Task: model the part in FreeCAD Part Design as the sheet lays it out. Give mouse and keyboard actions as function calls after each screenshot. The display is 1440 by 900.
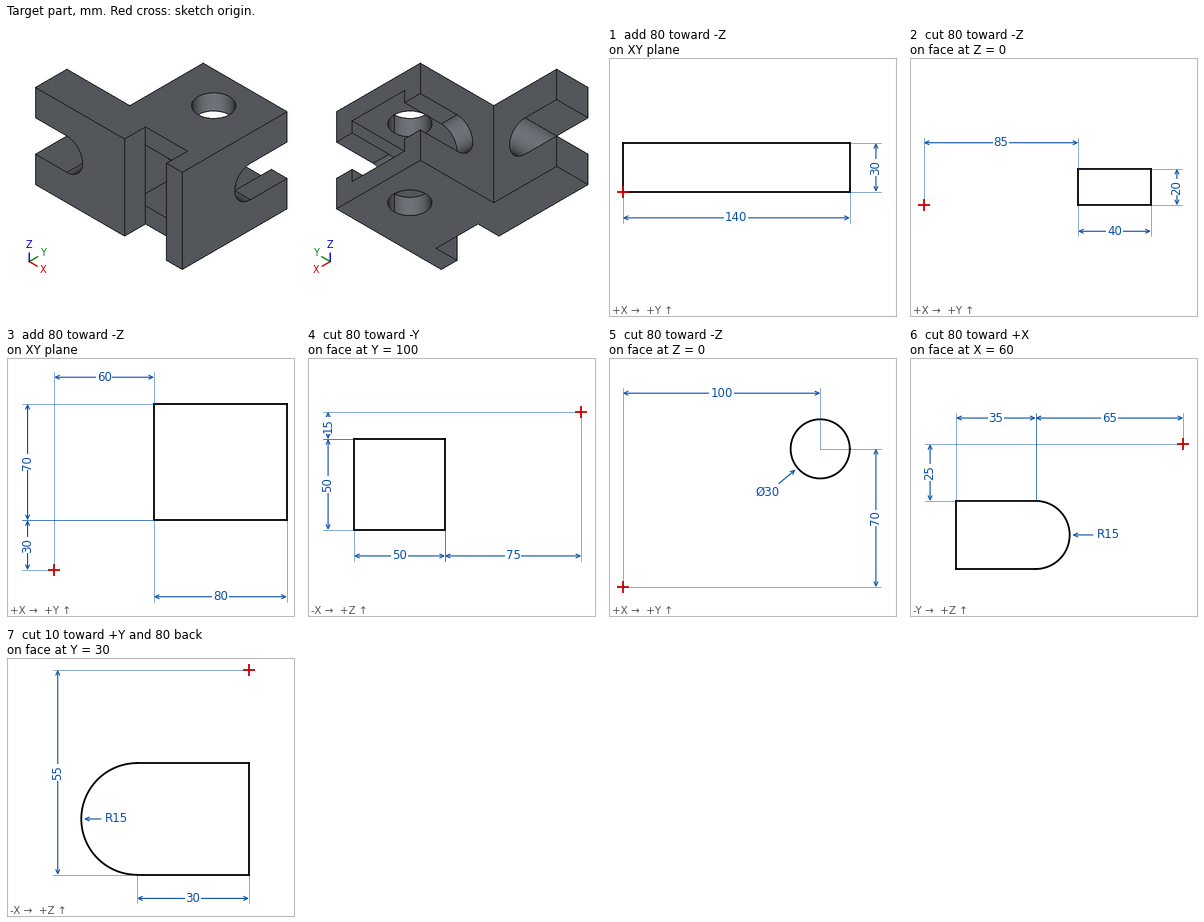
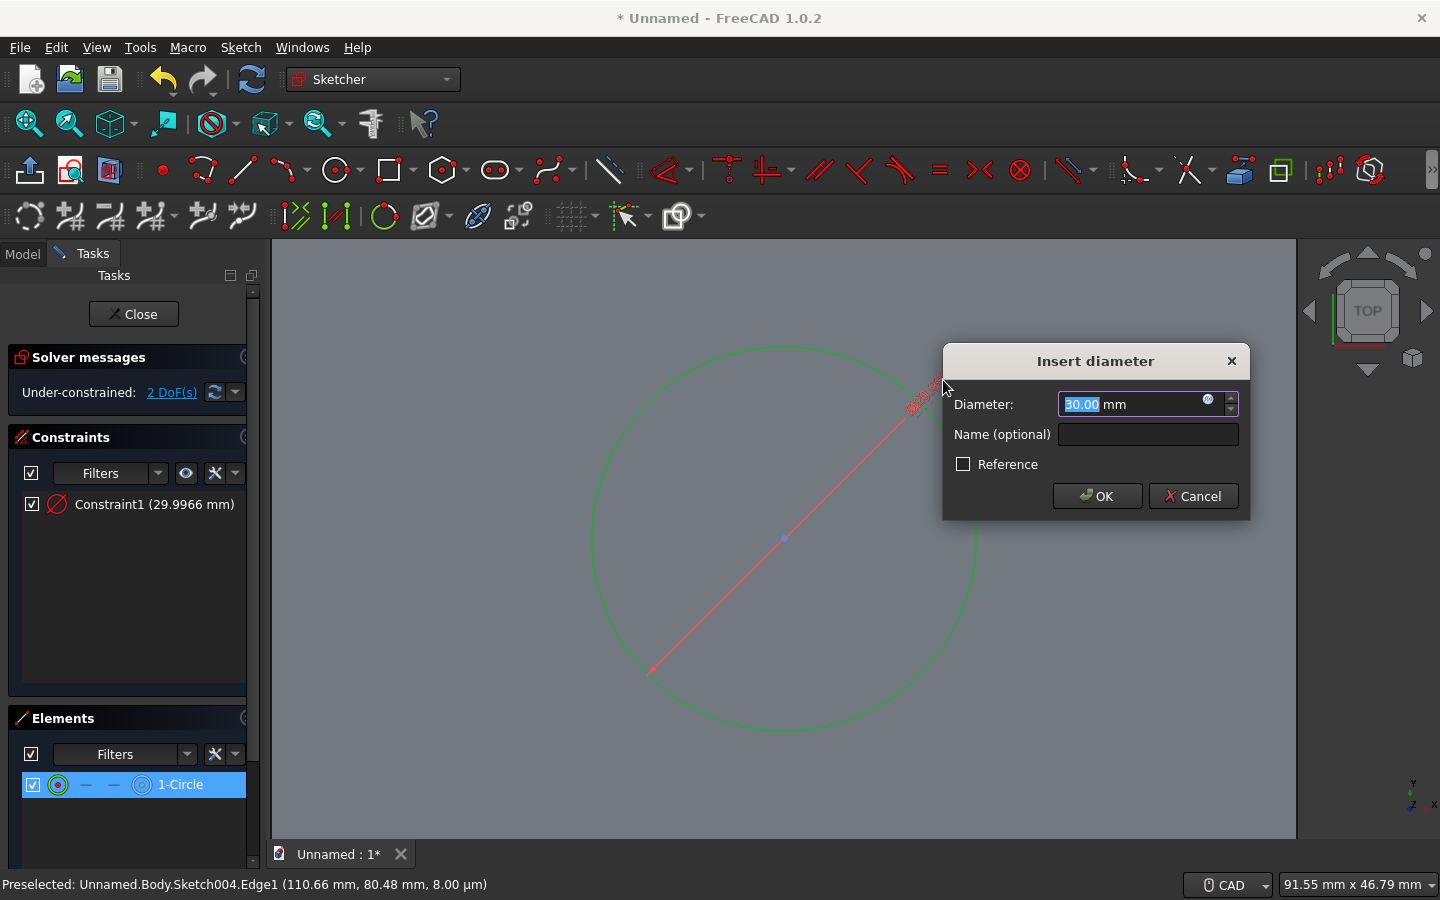
text(30)
key(Return)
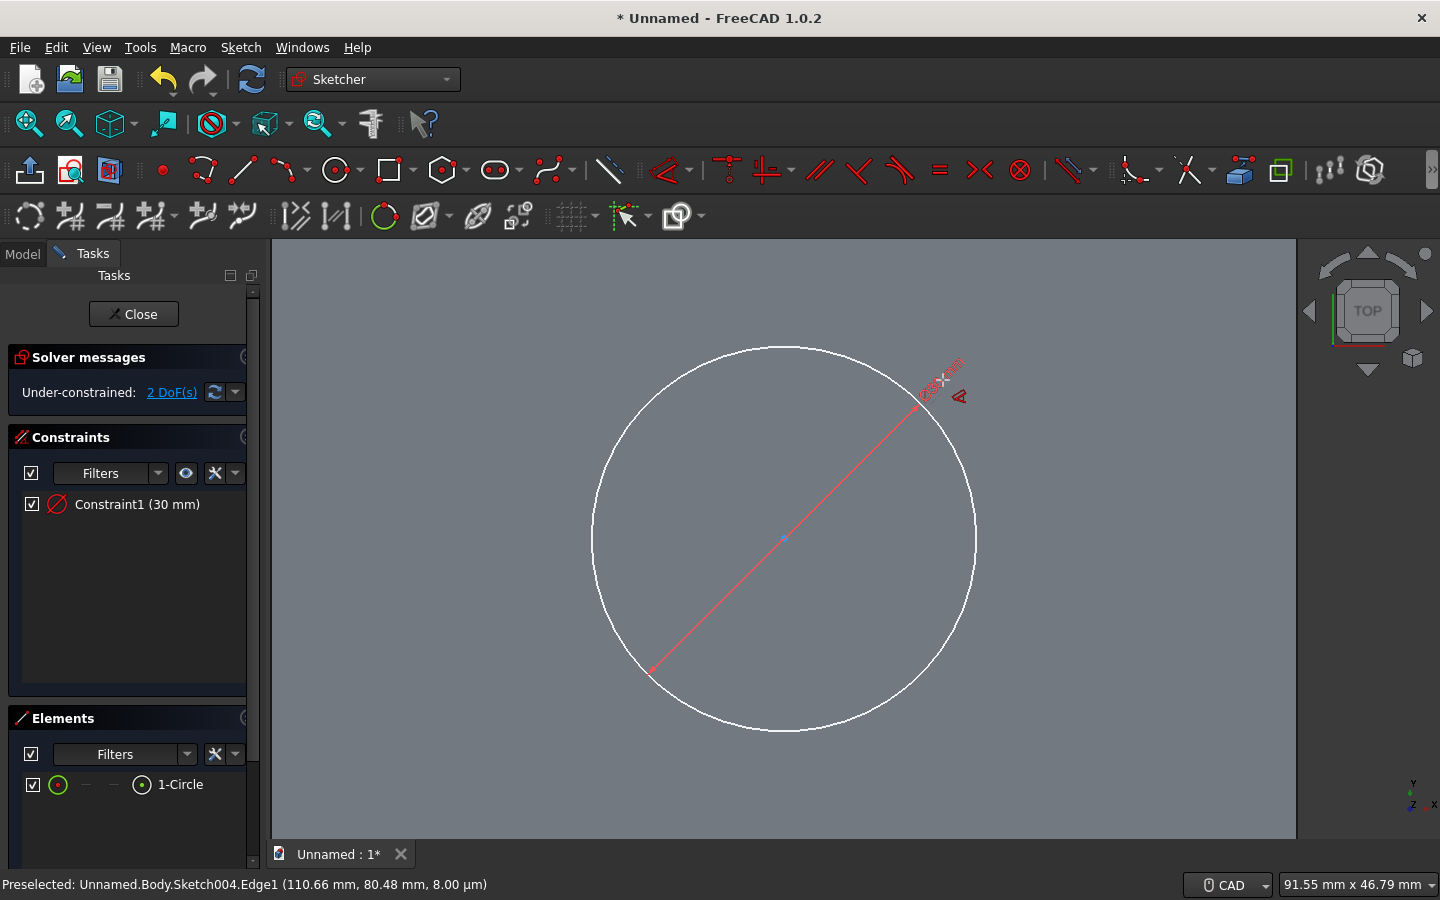
click(784, 539)
click(818, 675)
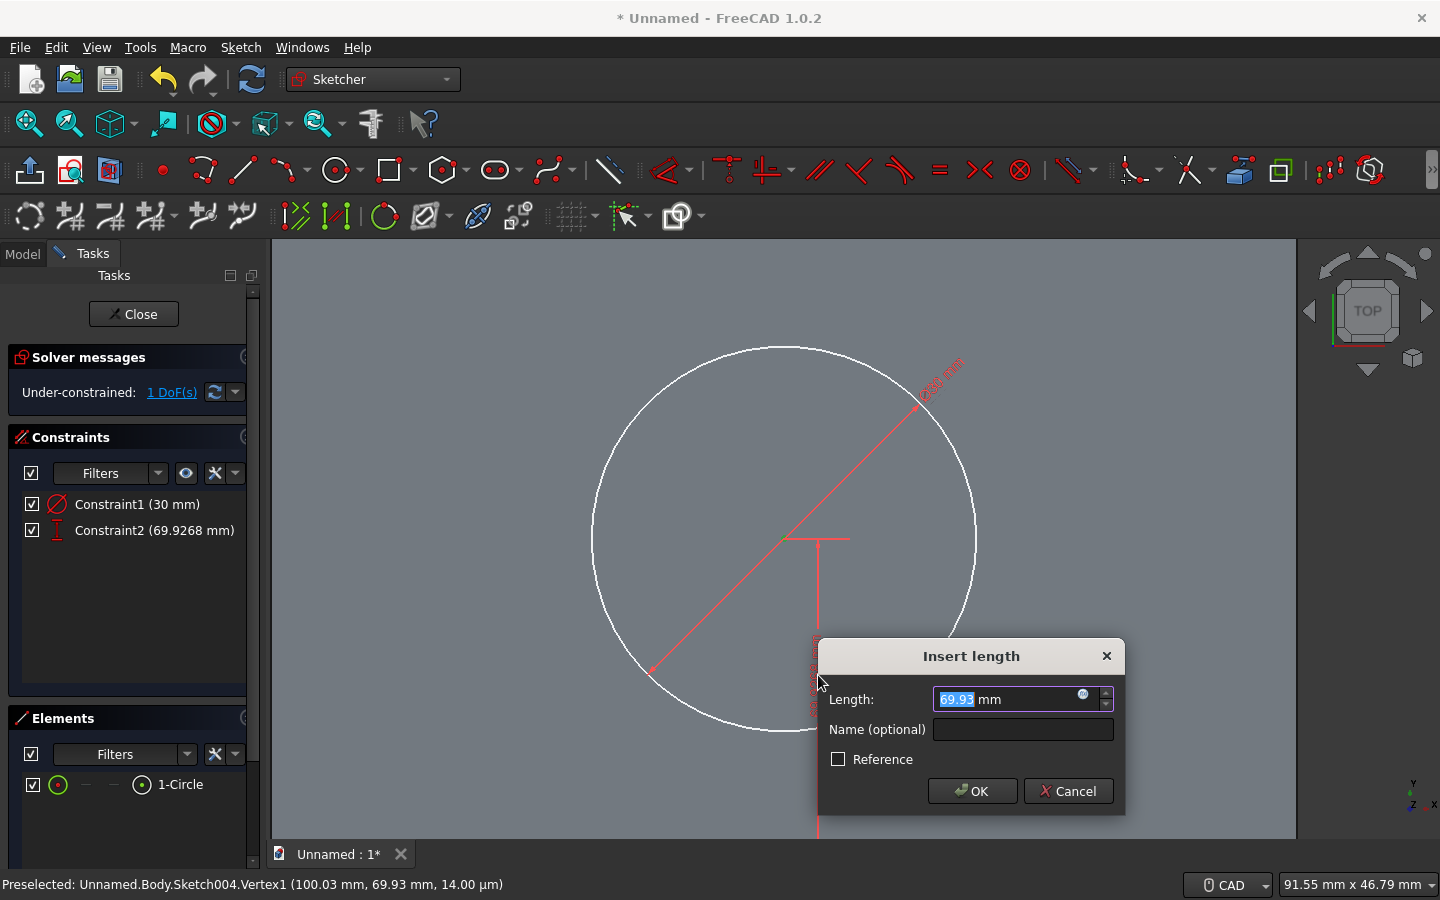
text(70)
key(Return)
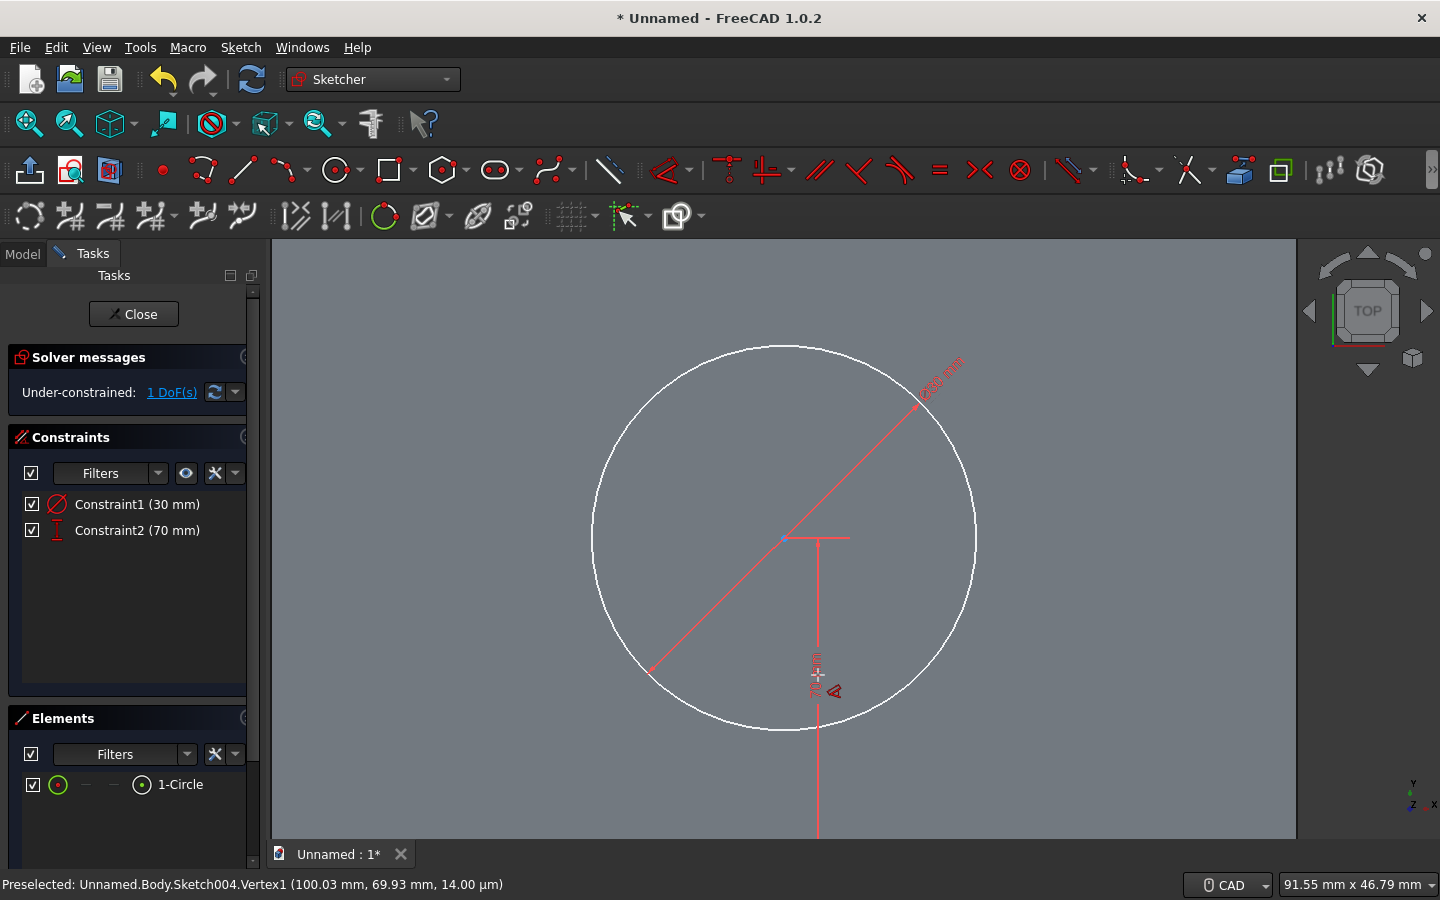
click(784, 538)
click(539, 504)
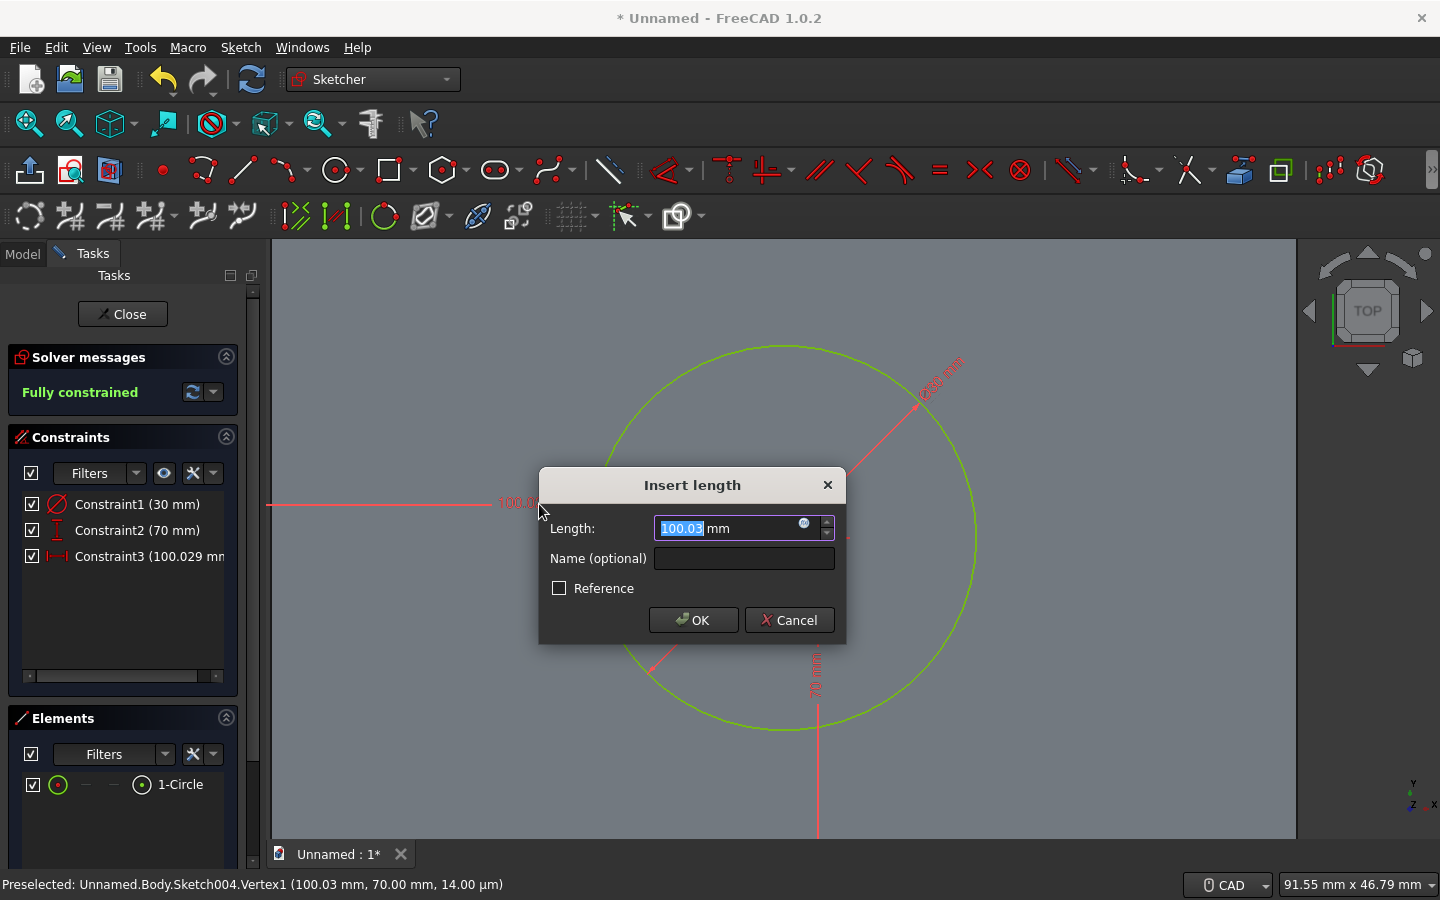
text(100)
key(Return)
key(Escape)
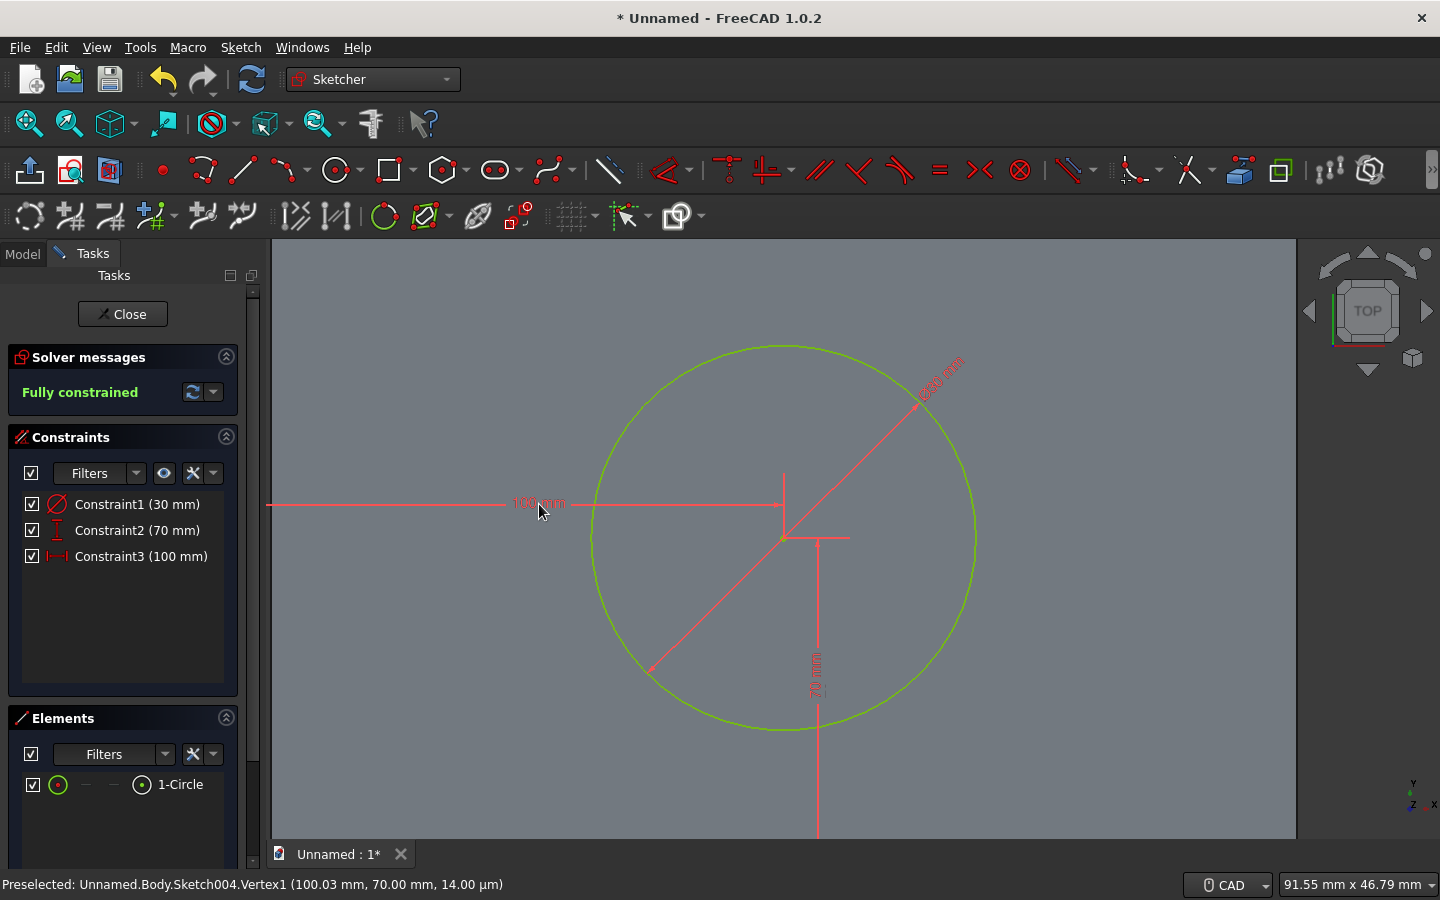
click(123, 314)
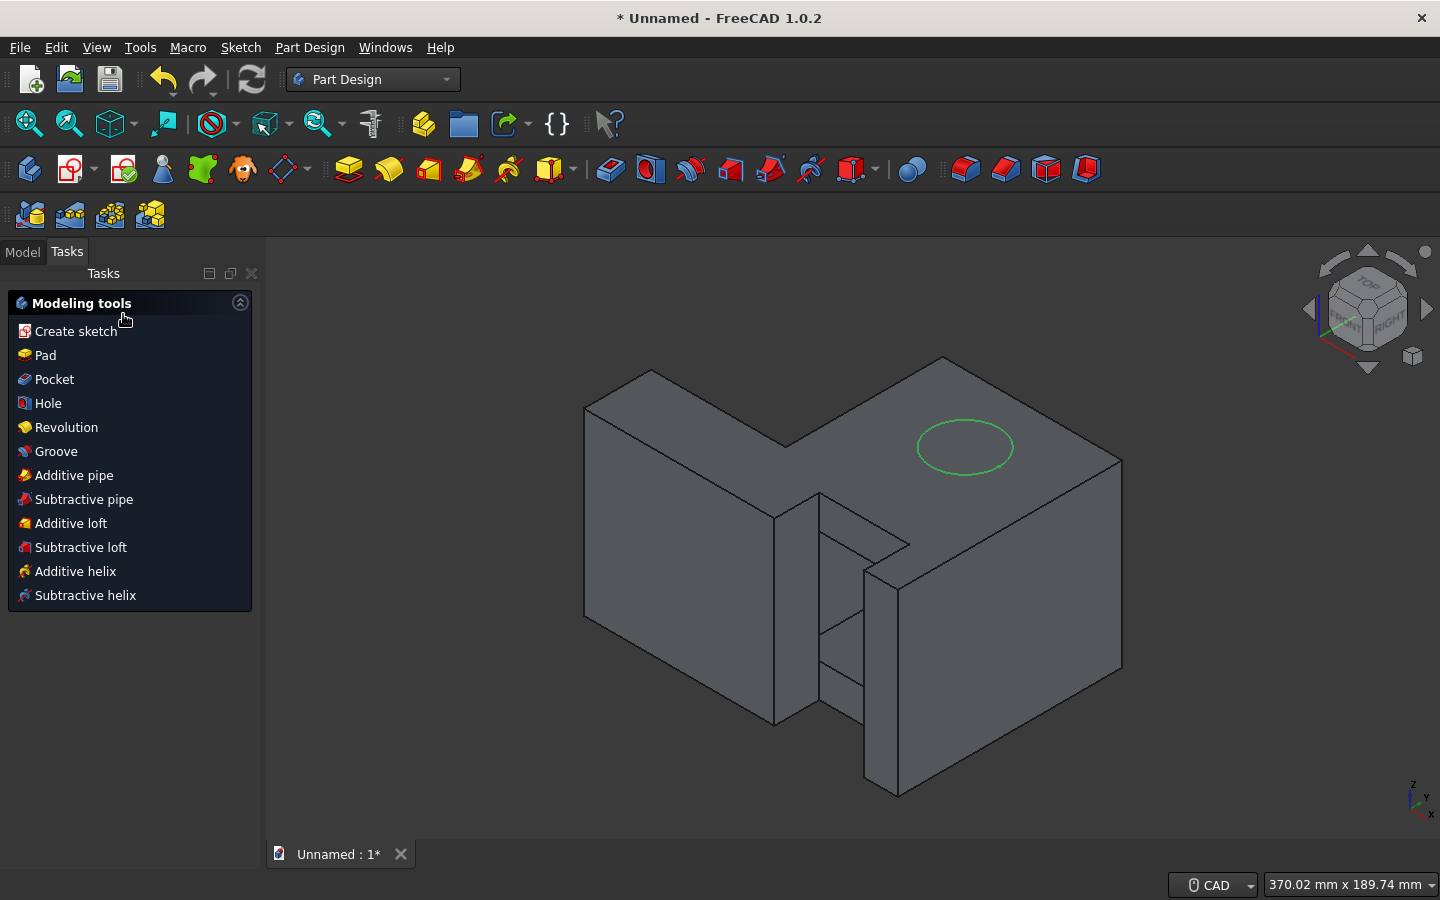
click(612, 170)